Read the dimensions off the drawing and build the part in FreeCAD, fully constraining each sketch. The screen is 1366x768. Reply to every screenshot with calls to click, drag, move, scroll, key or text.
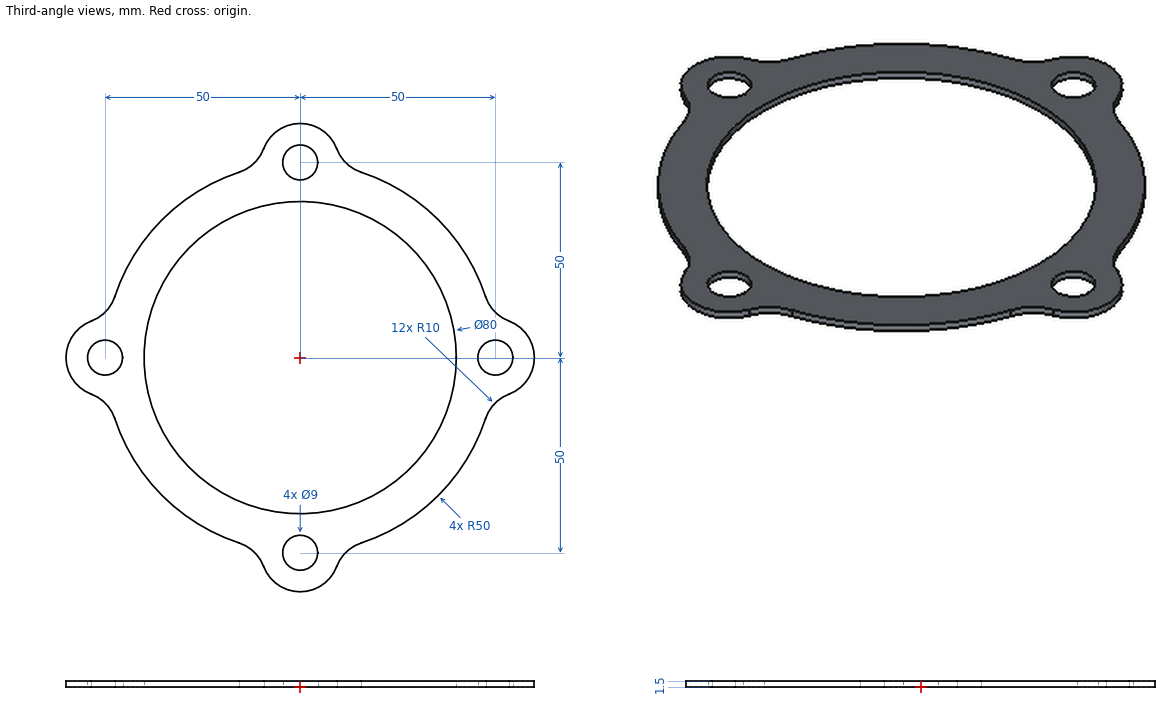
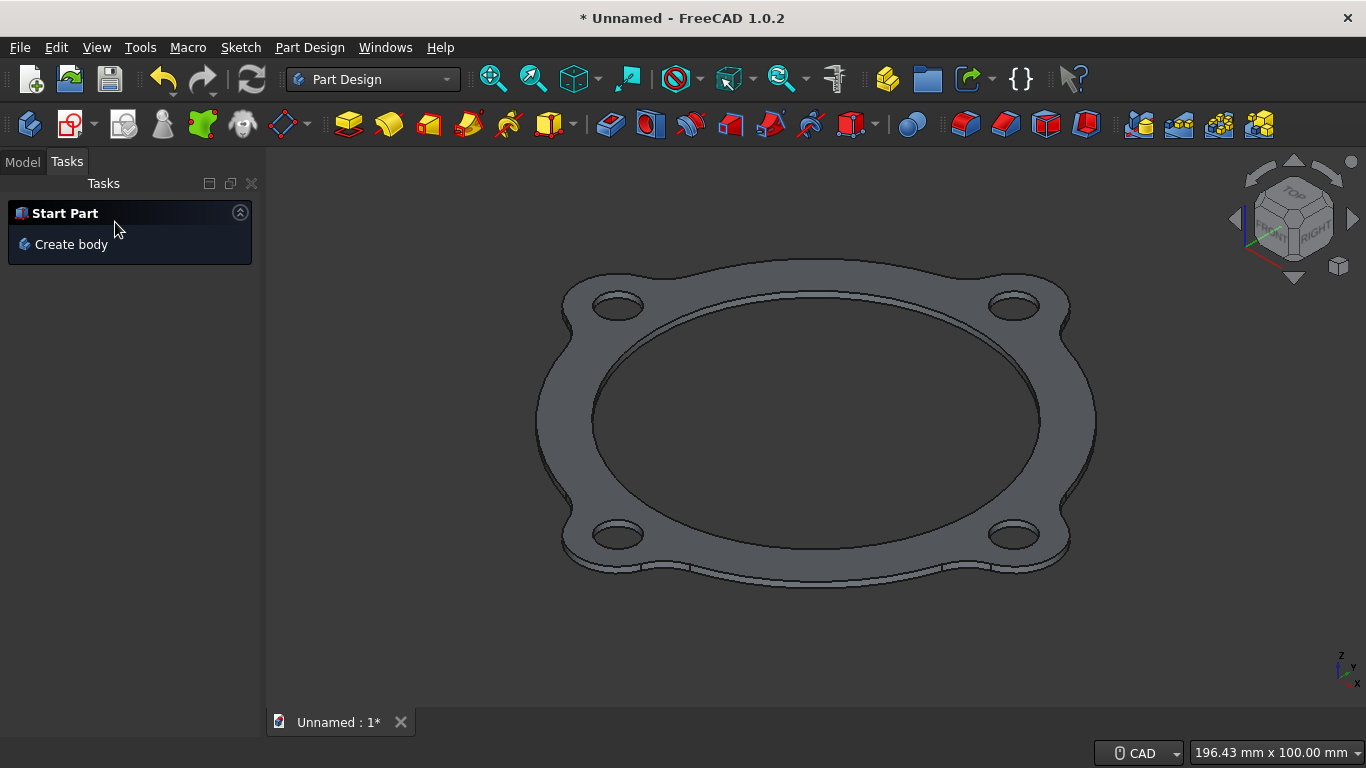
click(494, 80)